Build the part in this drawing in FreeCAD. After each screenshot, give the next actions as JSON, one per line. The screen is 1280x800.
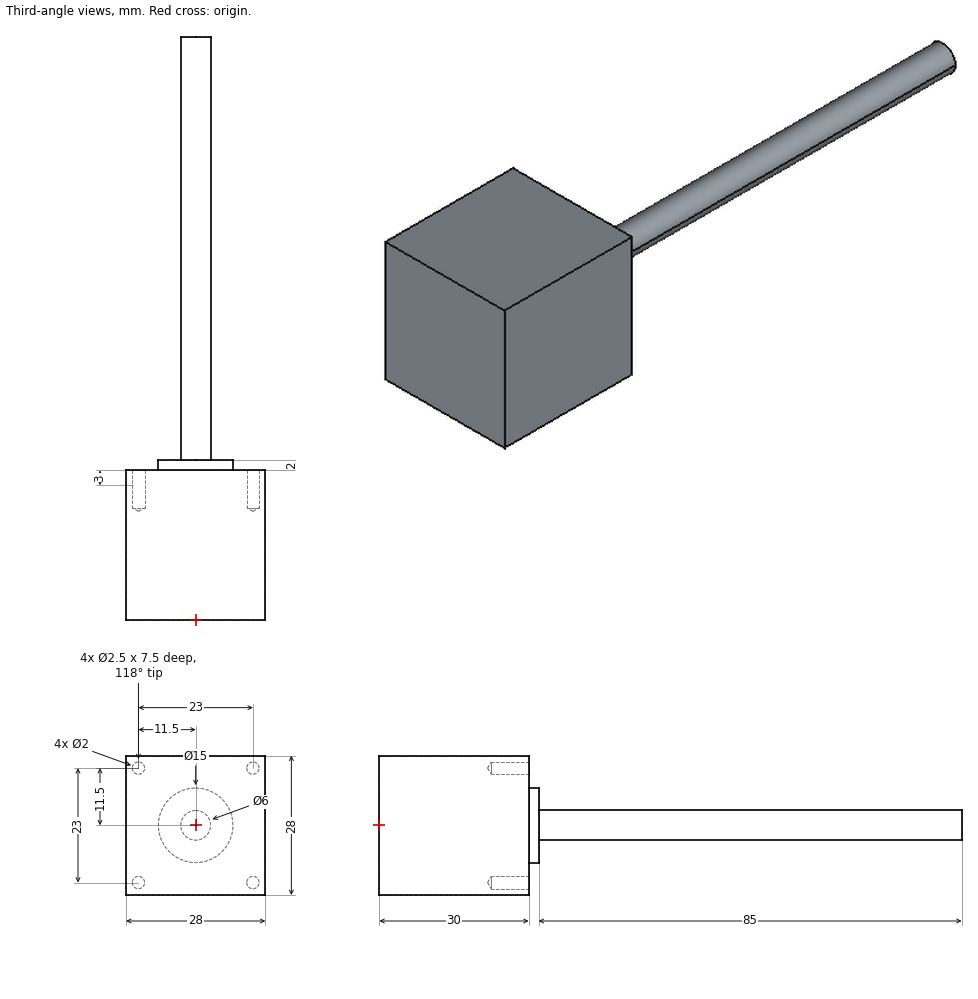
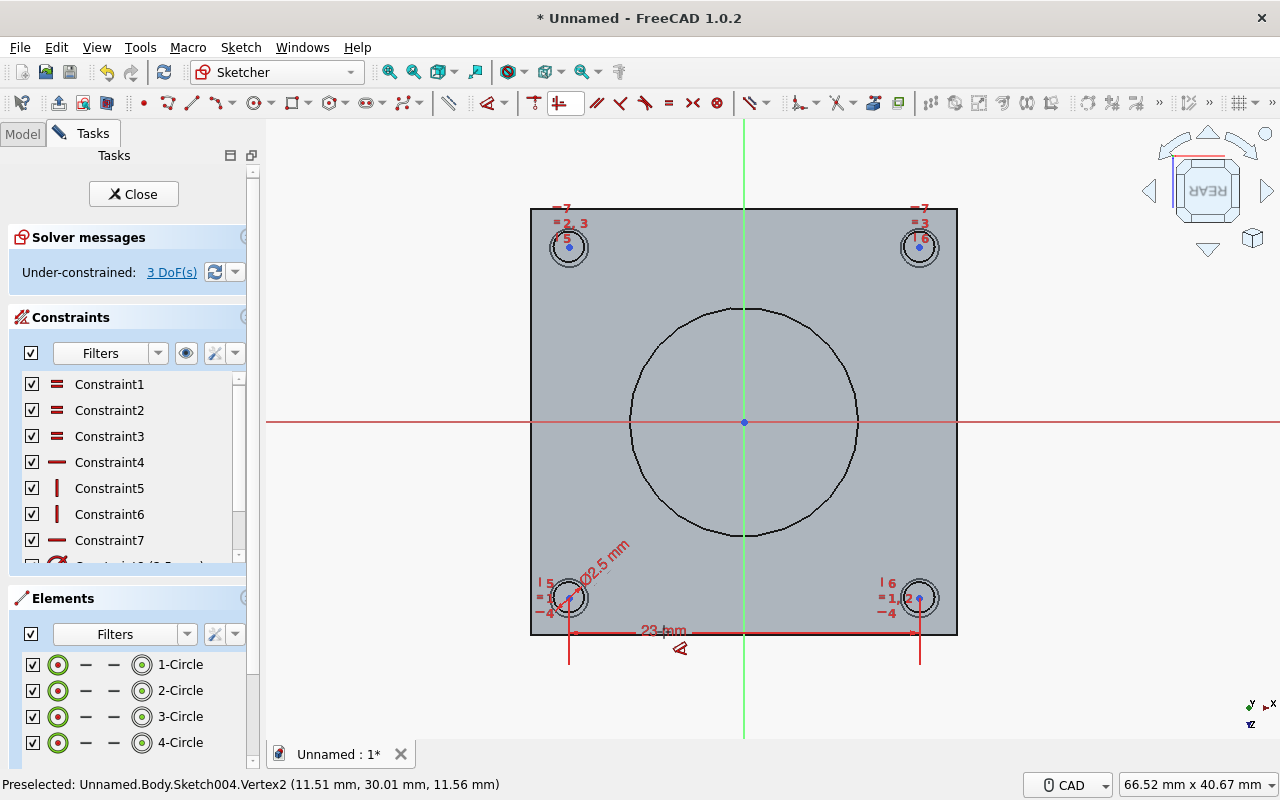
{"action": "left_click", "coordinate": [569, 598]}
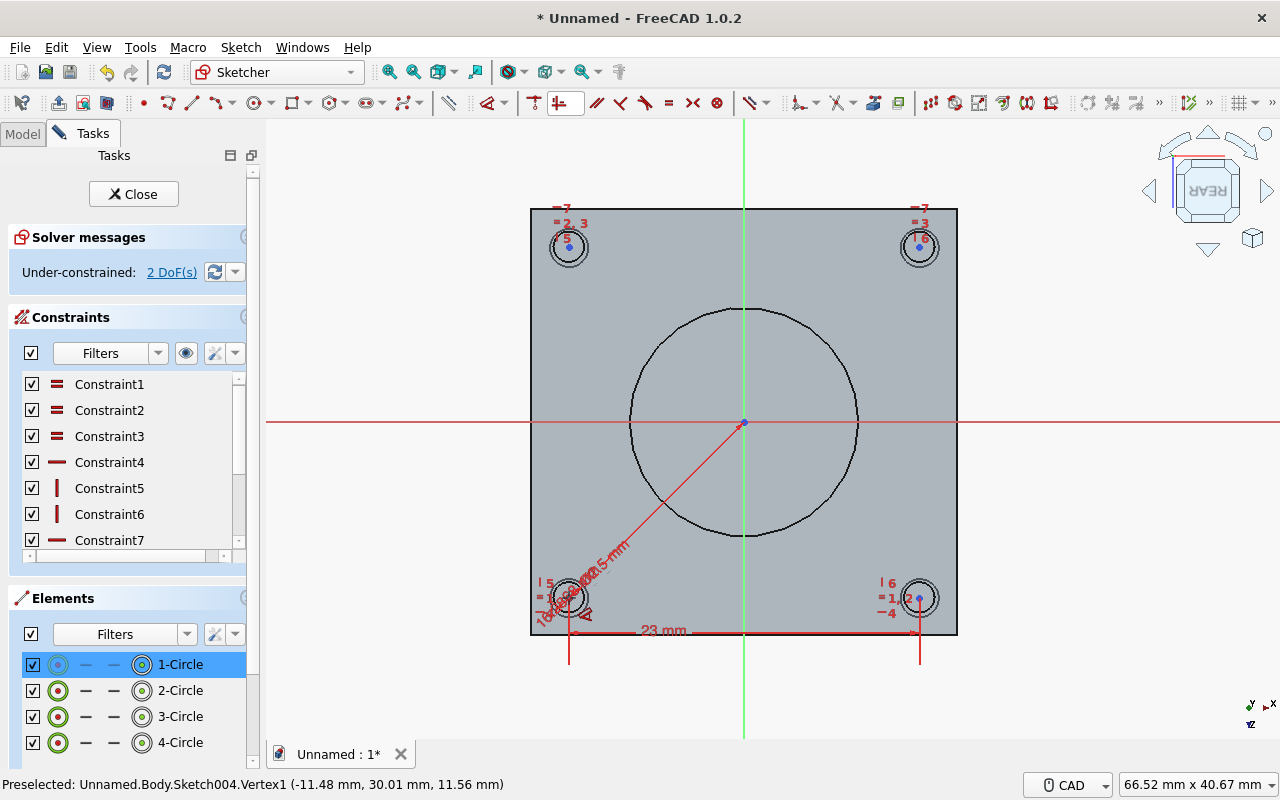
{"action": "left_click", "coordinate": [569, 248]}
{"action": "left_click", "coordinate": [535, 343]}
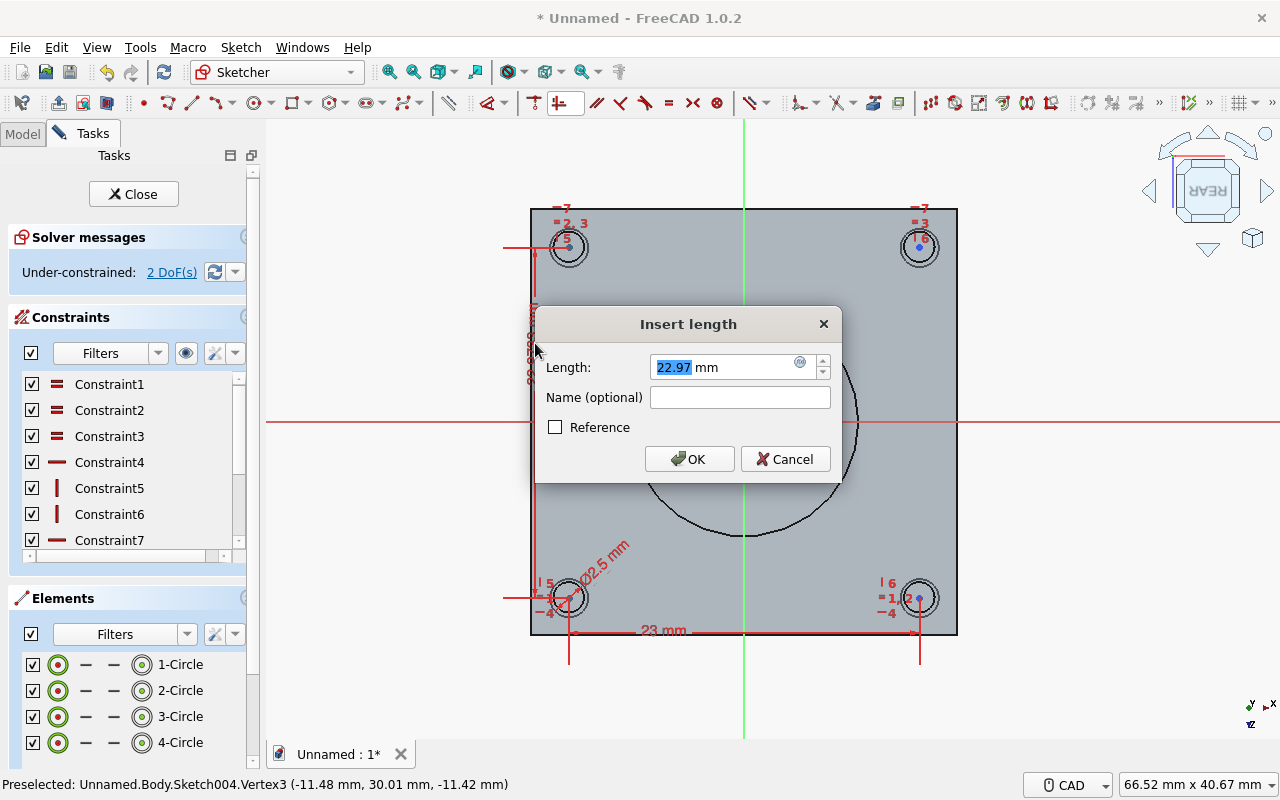
{"action": "type", "text": "23"}
{"action": "key", "text": "Return"}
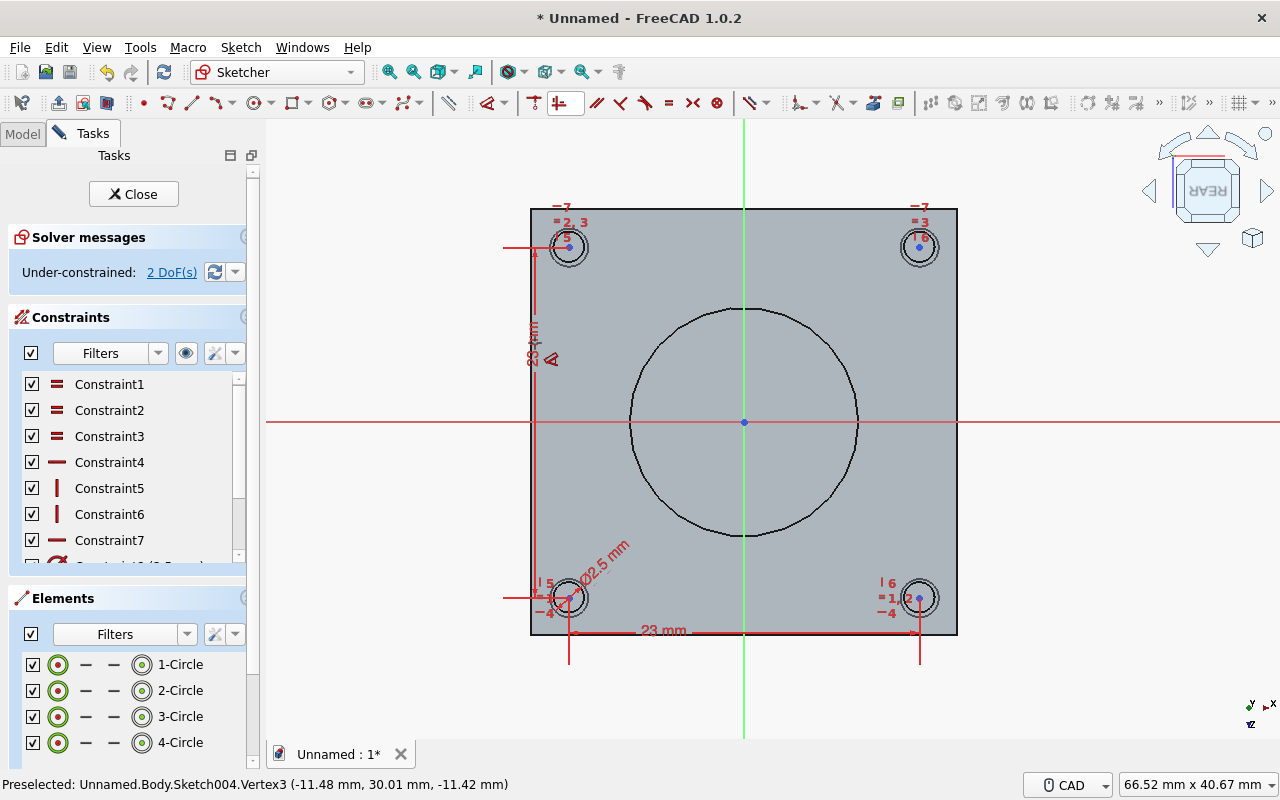
{"action": "left_click", "coordinate": [569, 598]}
{"action": "left_click", "coordinate": [657, 388]}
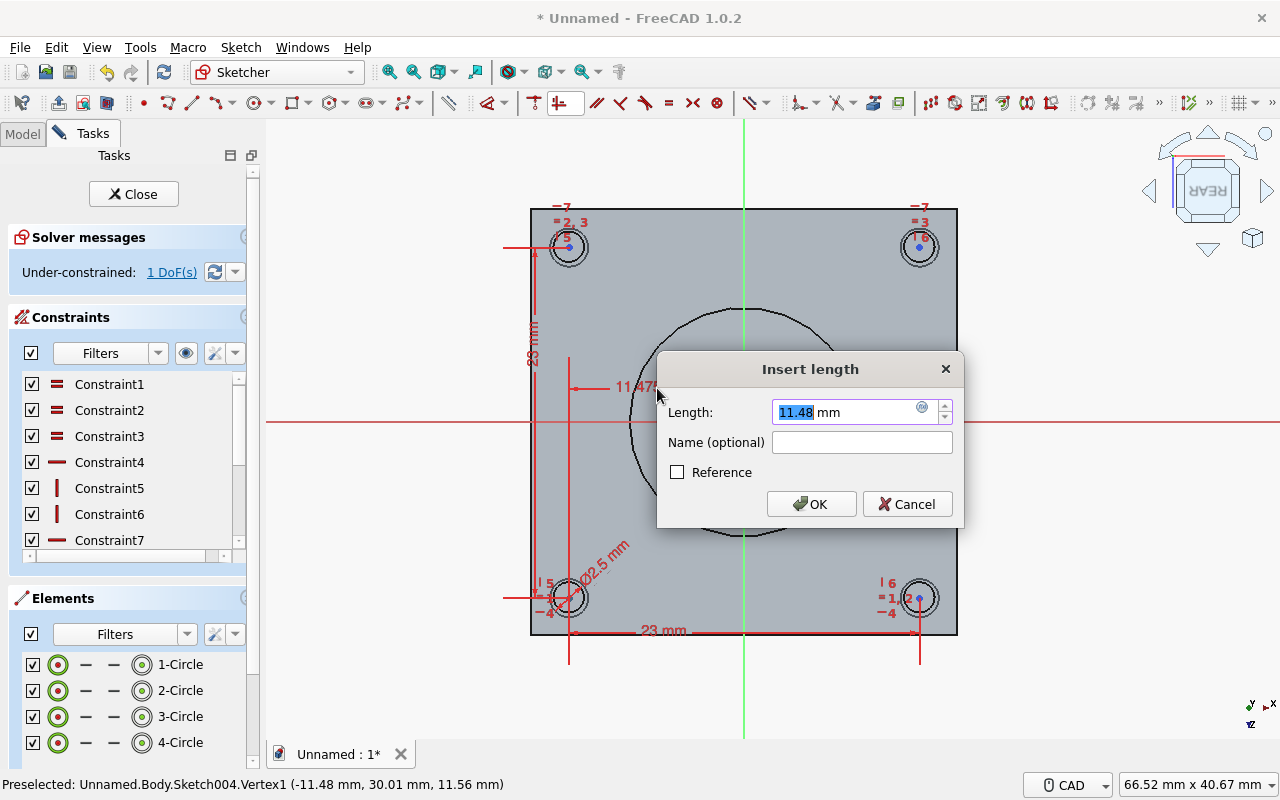
{"action": "type", "text": "11.5"}
{"action": "key", "text": "Return"}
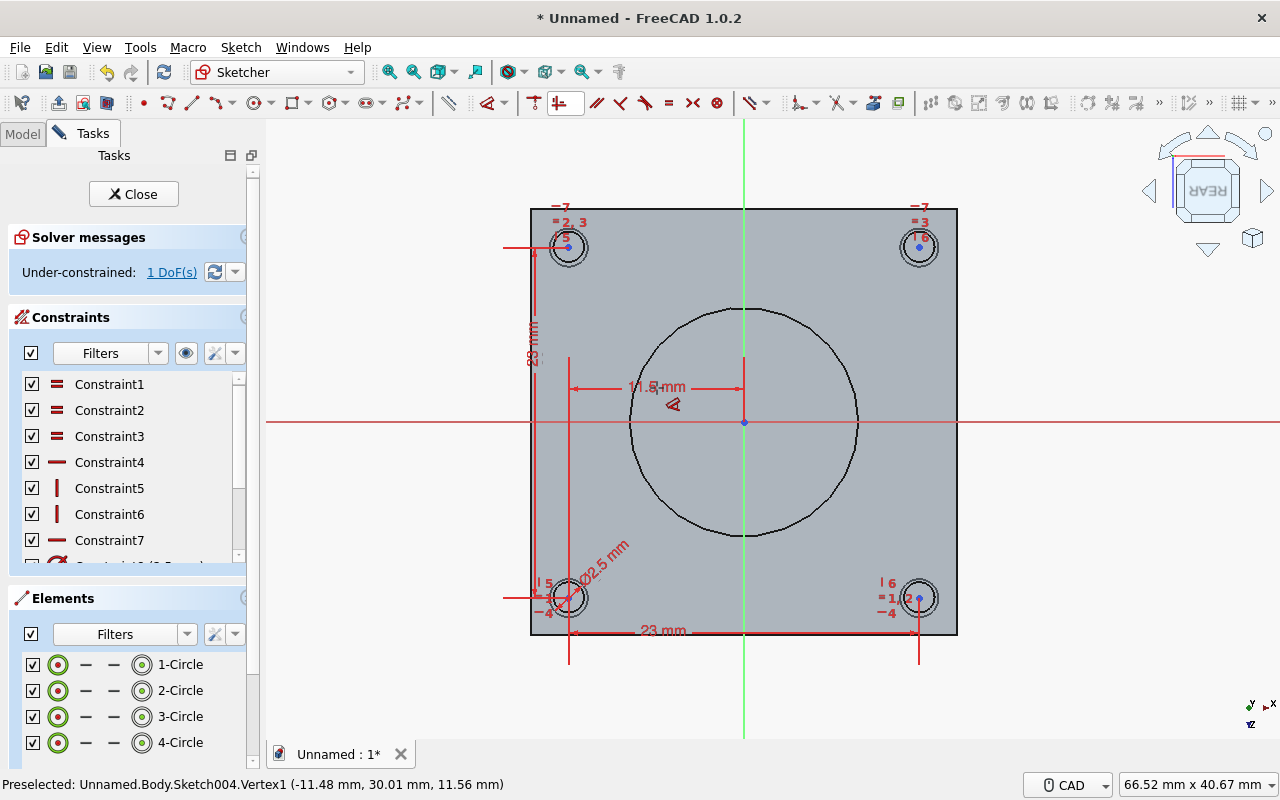
{"action": "left_click", "coordinate": [569, 598]}
{"action": "left_click", "coordinate": [535, 510]}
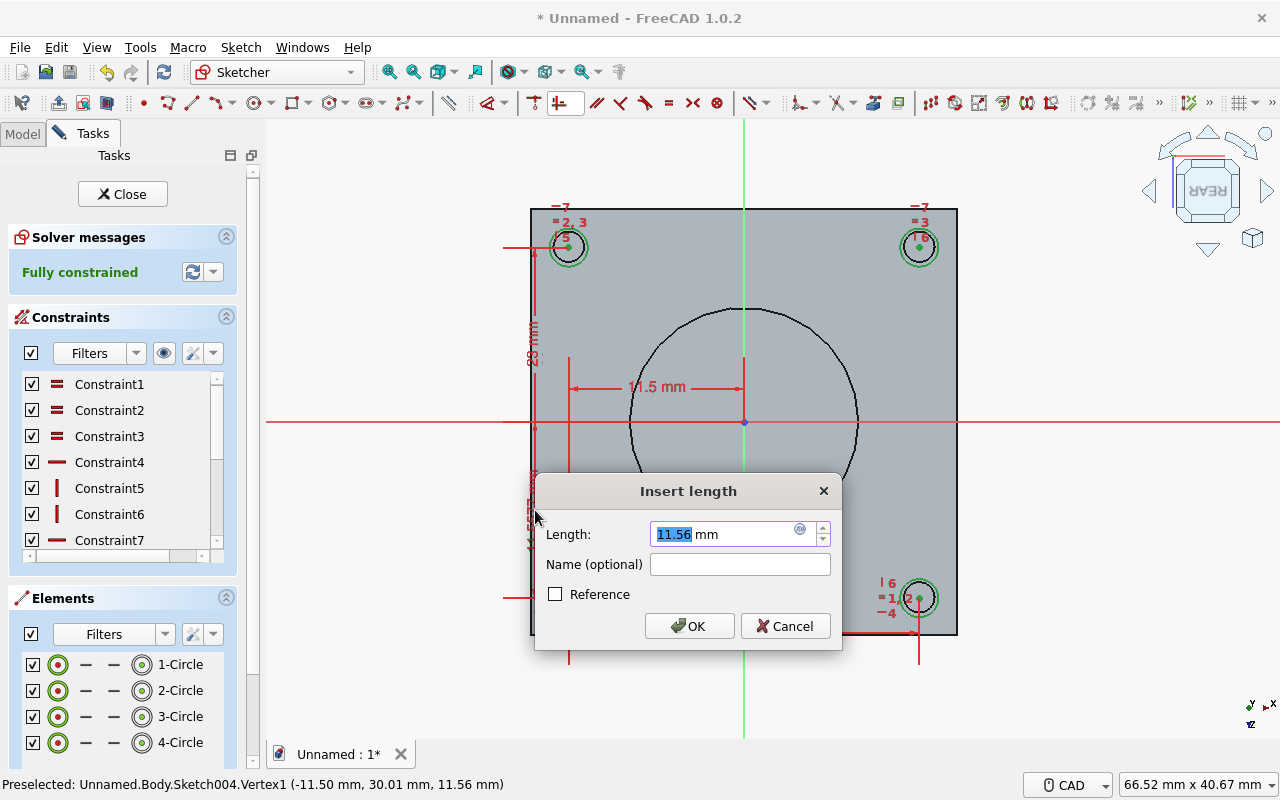
{"action": "type", "text": "11.5"}
{"action": "key", "text": "Return"}
{"action": "key", "text": "Escape"}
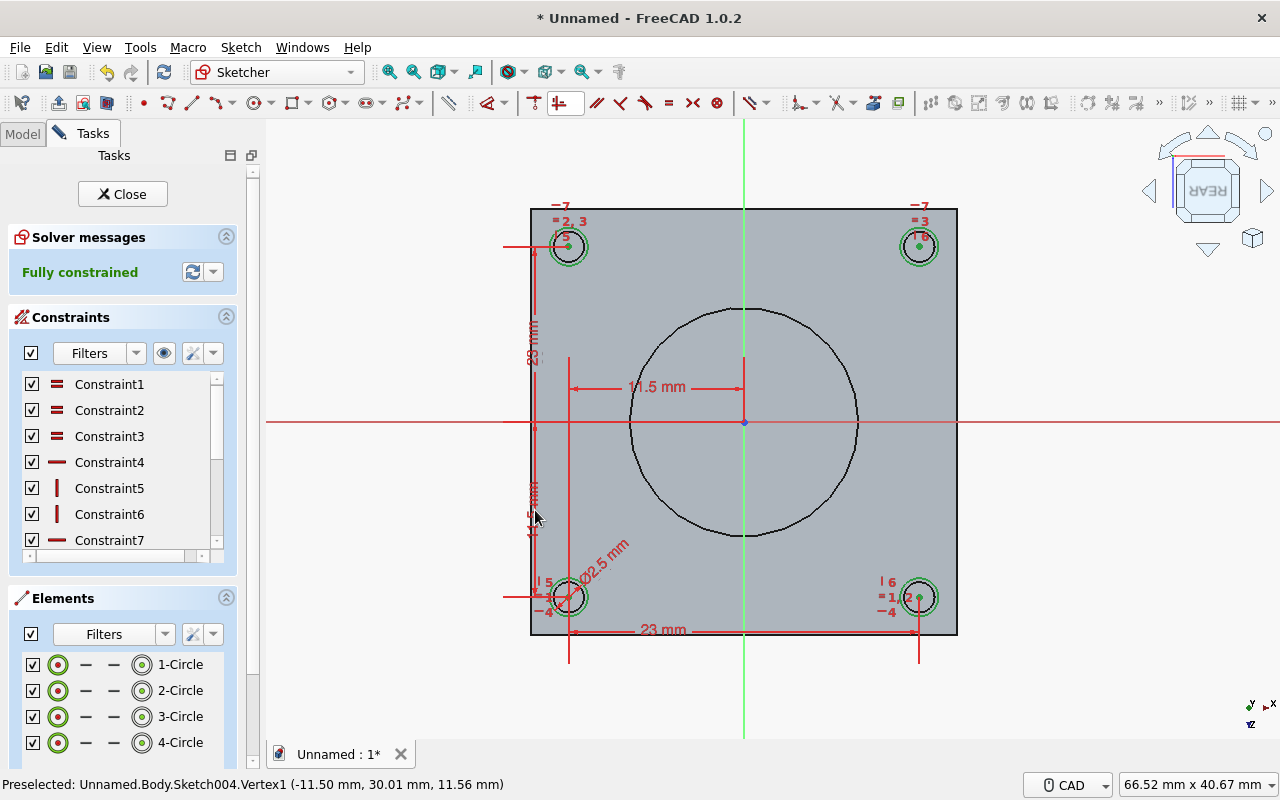
{"action": "left_click", "coordinate": [123, 194]}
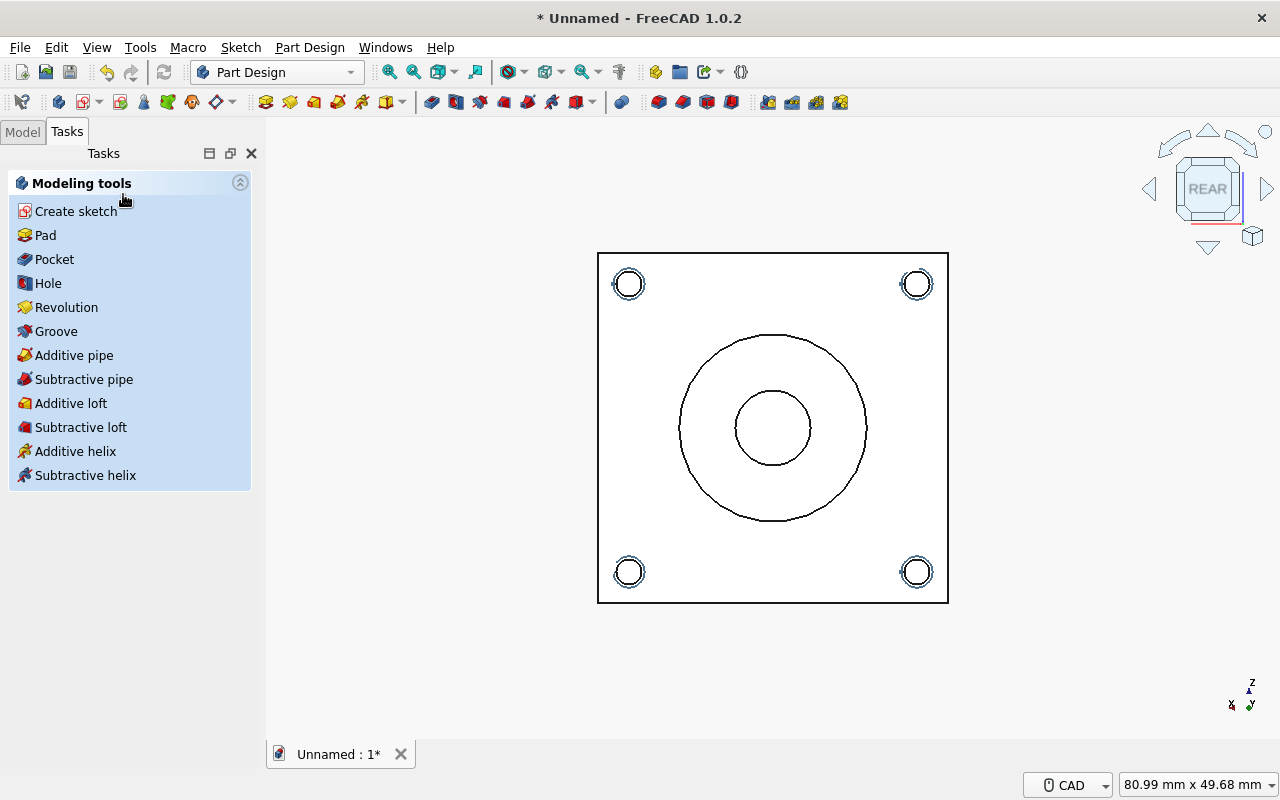
{"action": "left_click", "coordinate": [456, 102]}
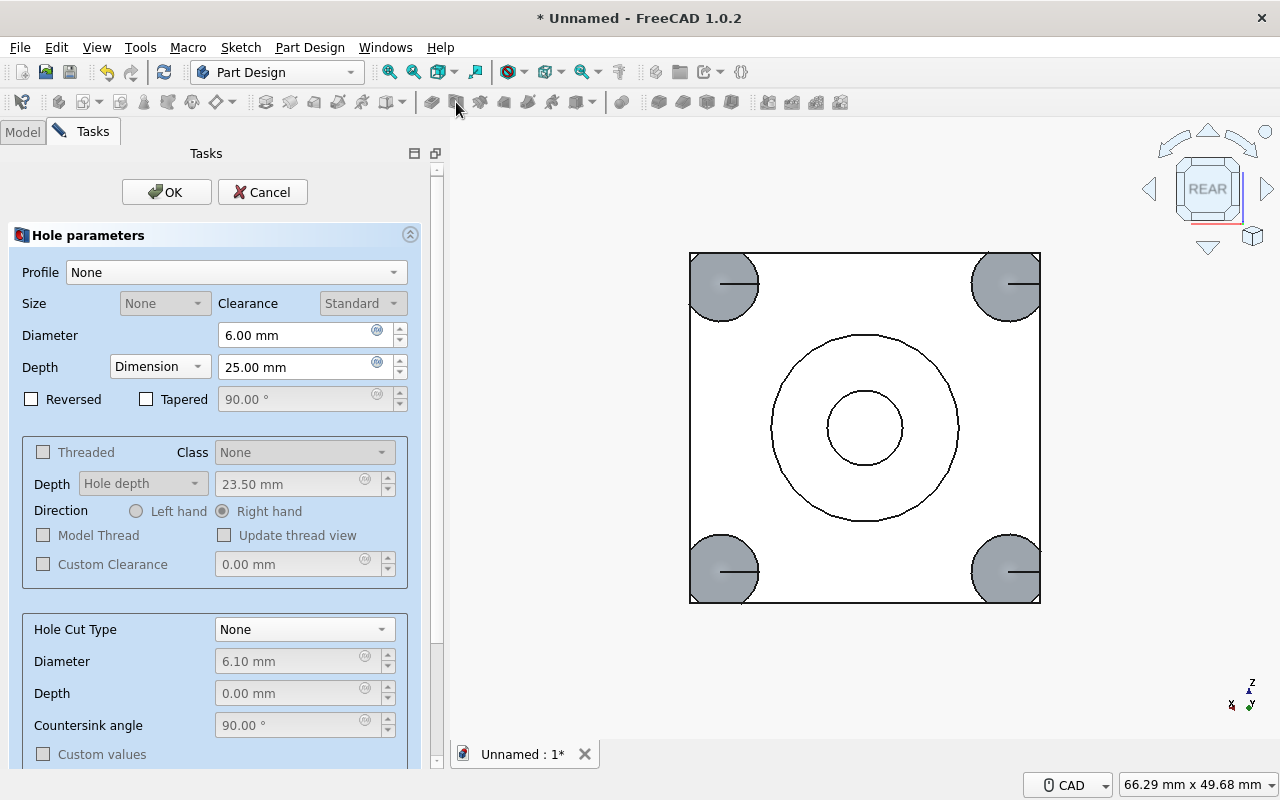
{"action": "triple_click", "coordinate": [305, 335]}